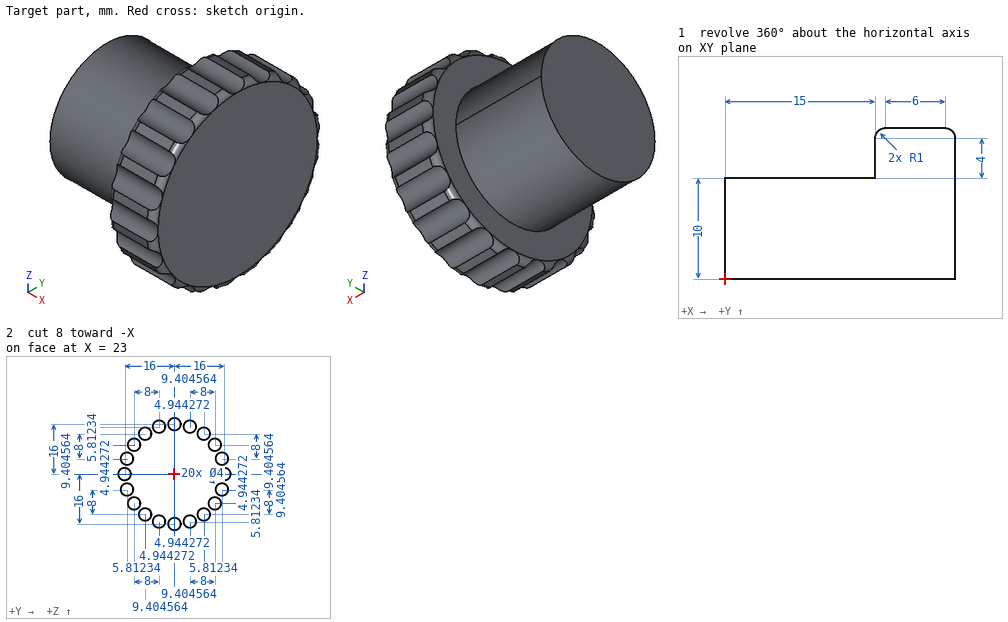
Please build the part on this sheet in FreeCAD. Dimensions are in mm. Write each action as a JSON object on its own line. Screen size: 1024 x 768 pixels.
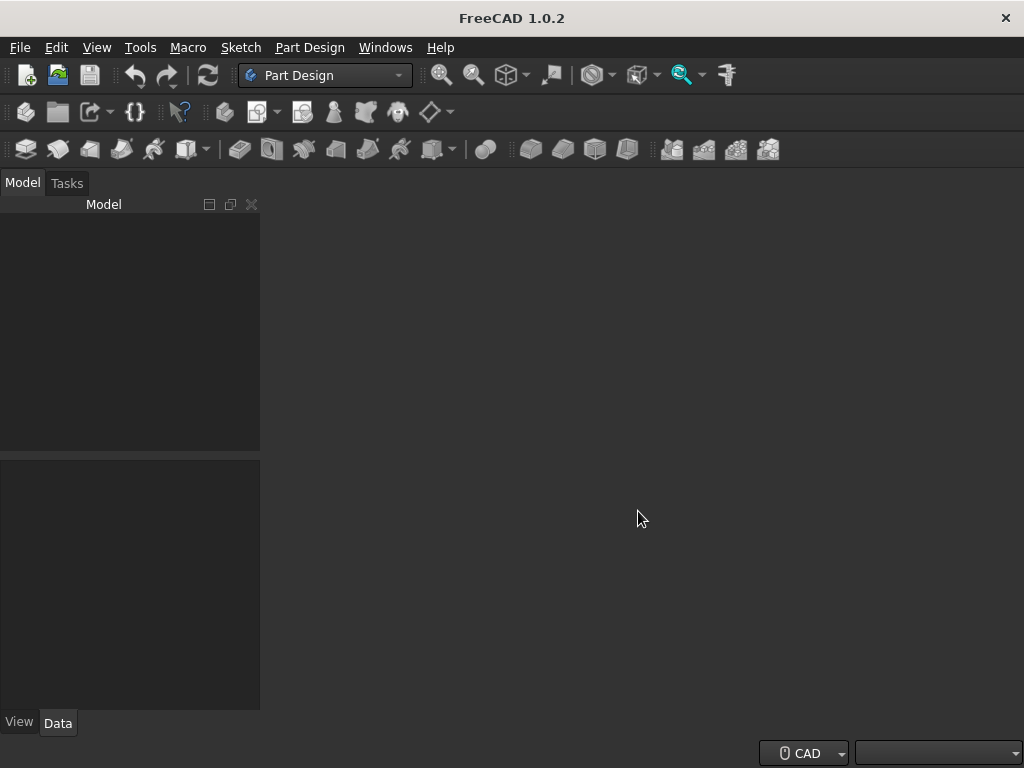
{"action": "left_click", "coordinate": [26, 76]}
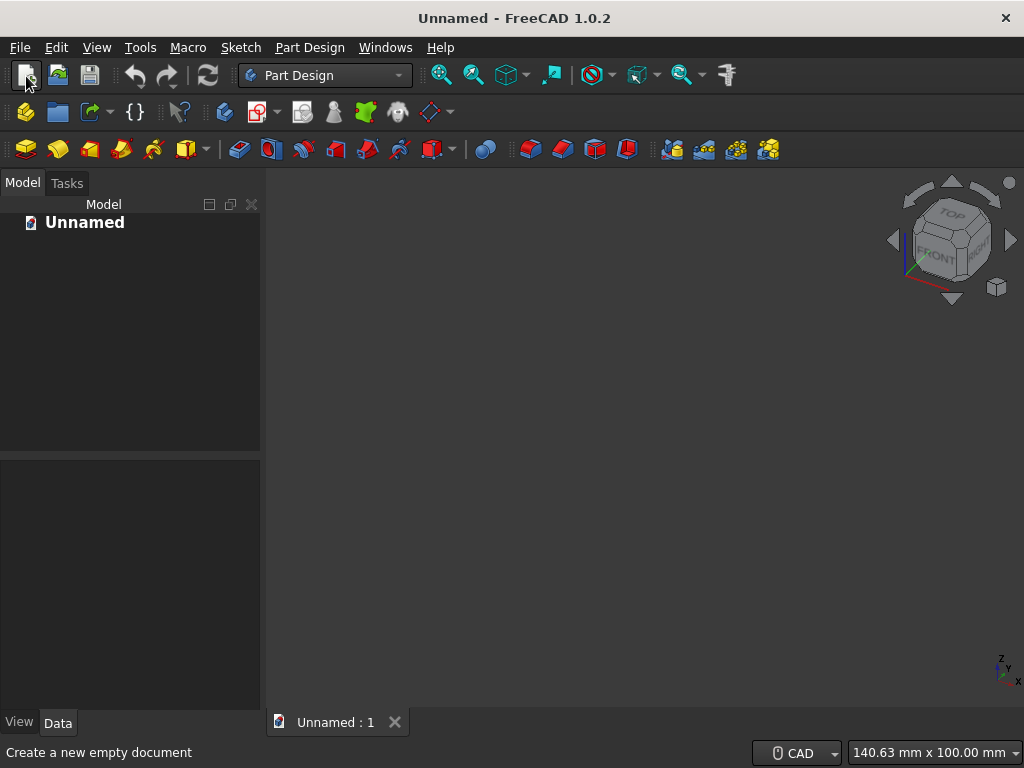
{"action": "left_click", "coordinate": [258, 112]}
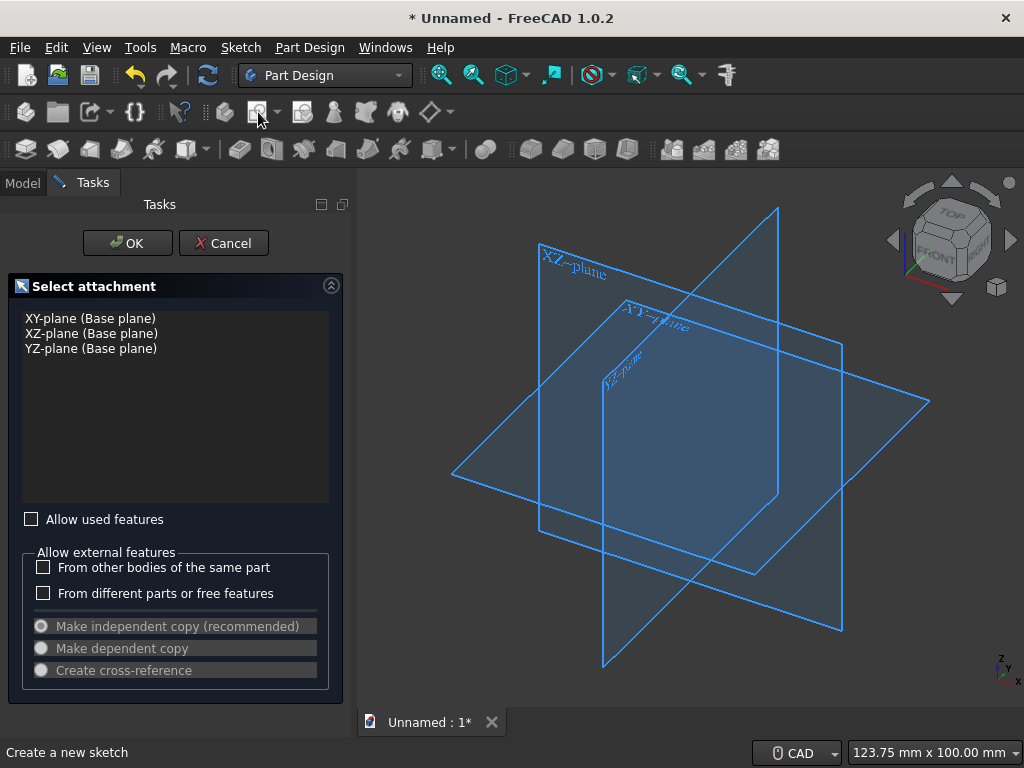
{"action": "left_click", "coordinate": [82, 318]}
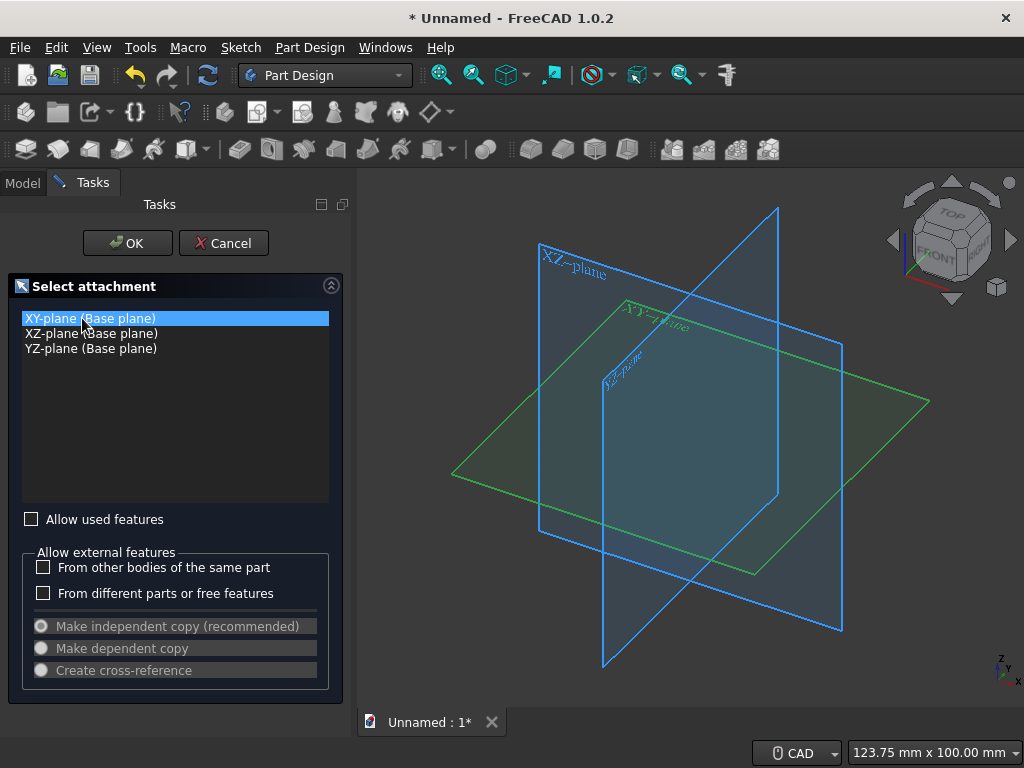
{"action": "left_click", "coordinate": [128, 243]}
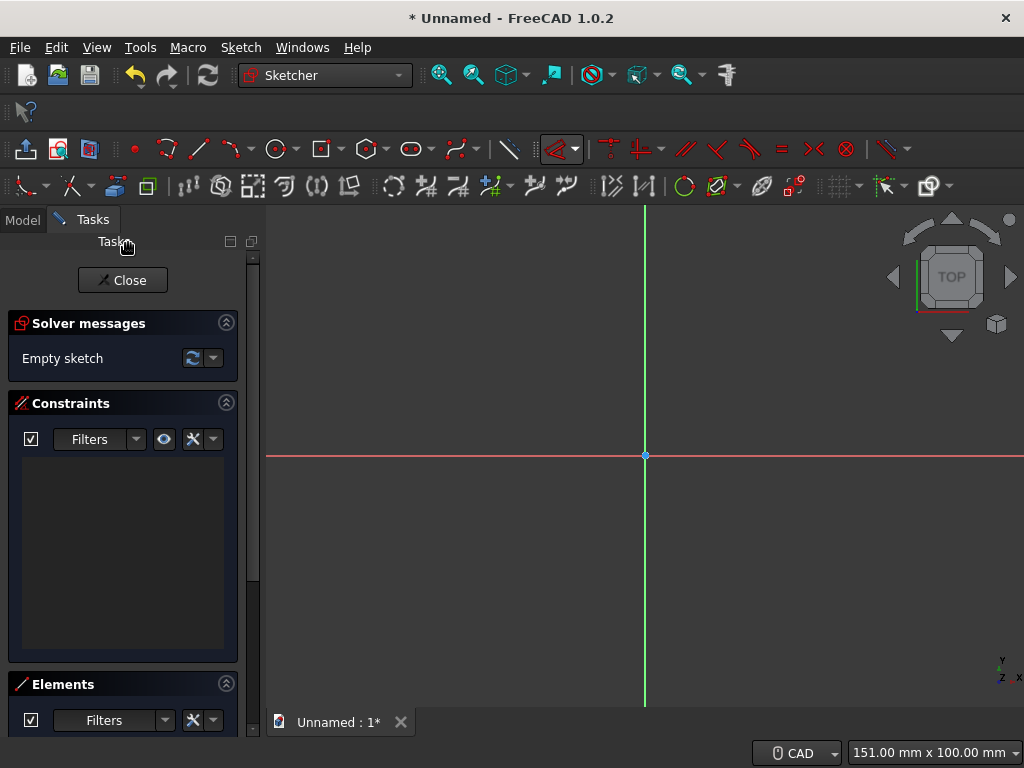
{"action": "scroll", "coordinate": [757, 402], "scroll_direction": "up", "scroll_amount": 6}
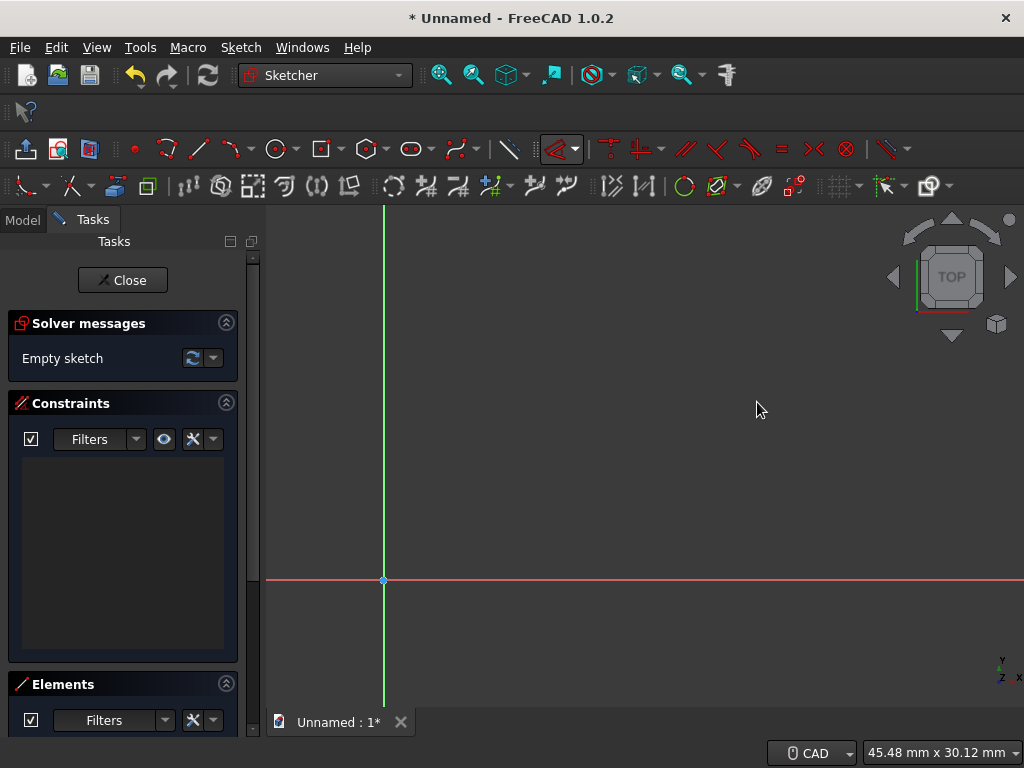
{"action": "left_click", "coordinate": [200, 150]}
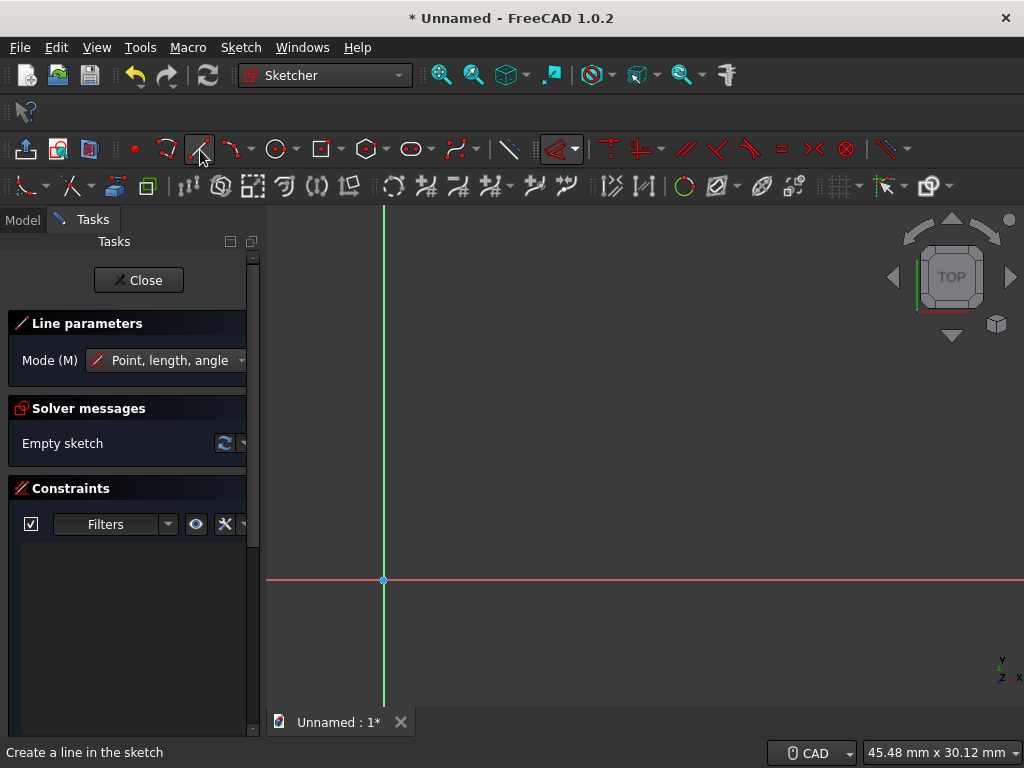
{"action": "left_click", "coordinate": [750, 330]}
{"action": "left_click", "coordinate": [650, 330]}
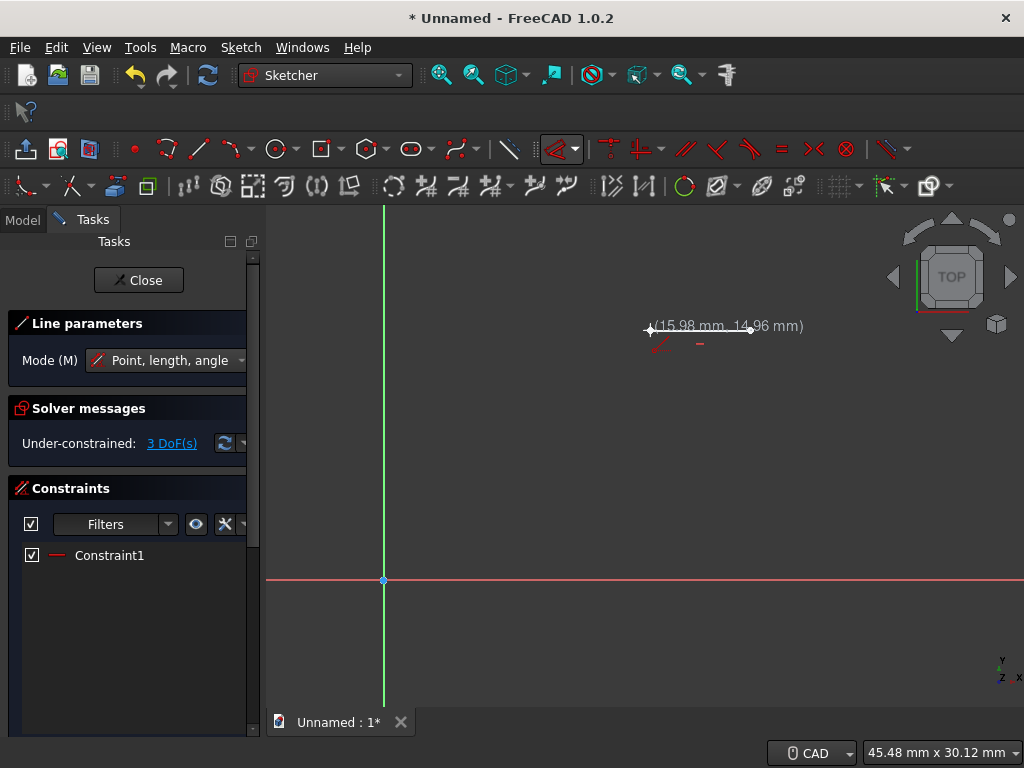
{"action": "left_click", "coordinate": [168, 150]}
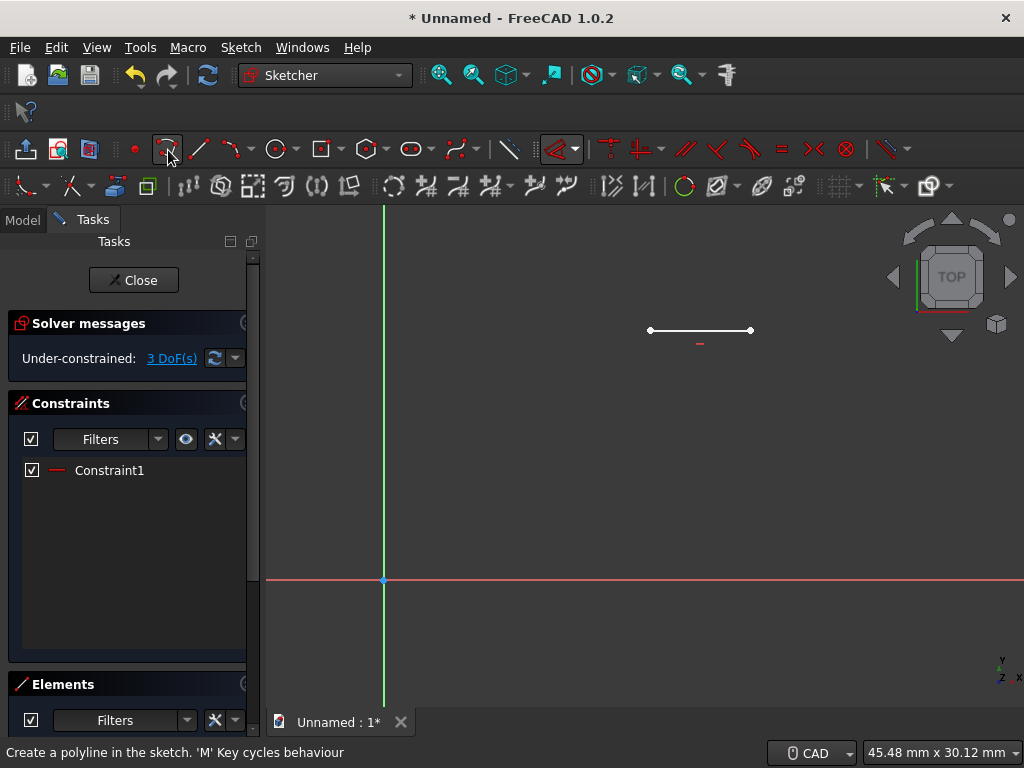
{"action": "left_click", "coordinate": [634, 347]}
{"action": "left_click", "coordinate": [634, 414]}
{"action": "left_click", "coordinate": [384, 414]}
{"action": "left_click", "coordinate": [384, 580]}
{"action": "left_click", "coordinate": [767, 571]}
{"action": "left_click", "coordinate": [767, 347]}
{"action": "right_click", "coordinate": [767, 347]}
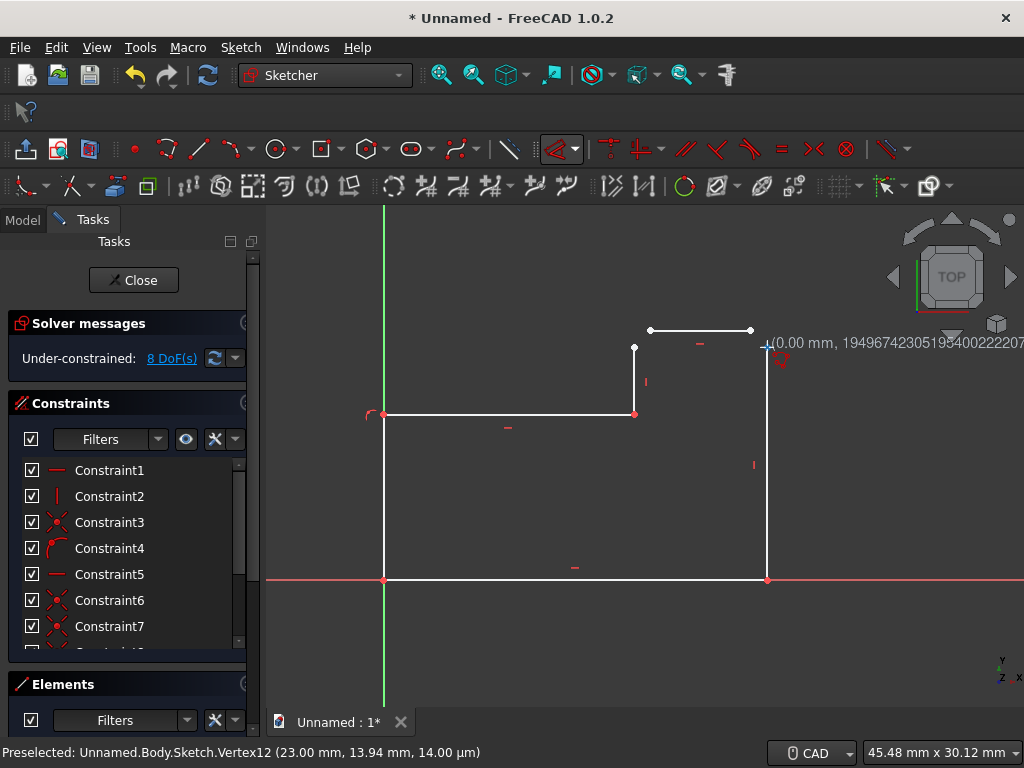
{"action": "left_click", "coordinate": [232, 150]}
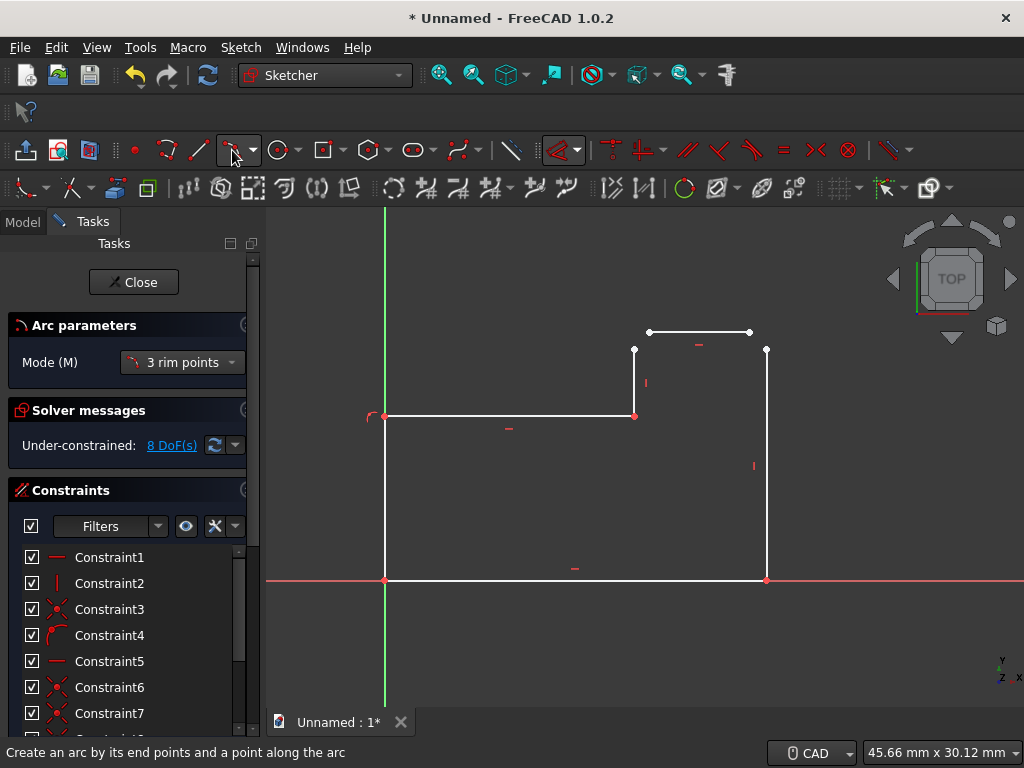
{"action": "left_click", "coordinate": [650, 332]}
{"action": "left_click", "coordinate": [634, 349]}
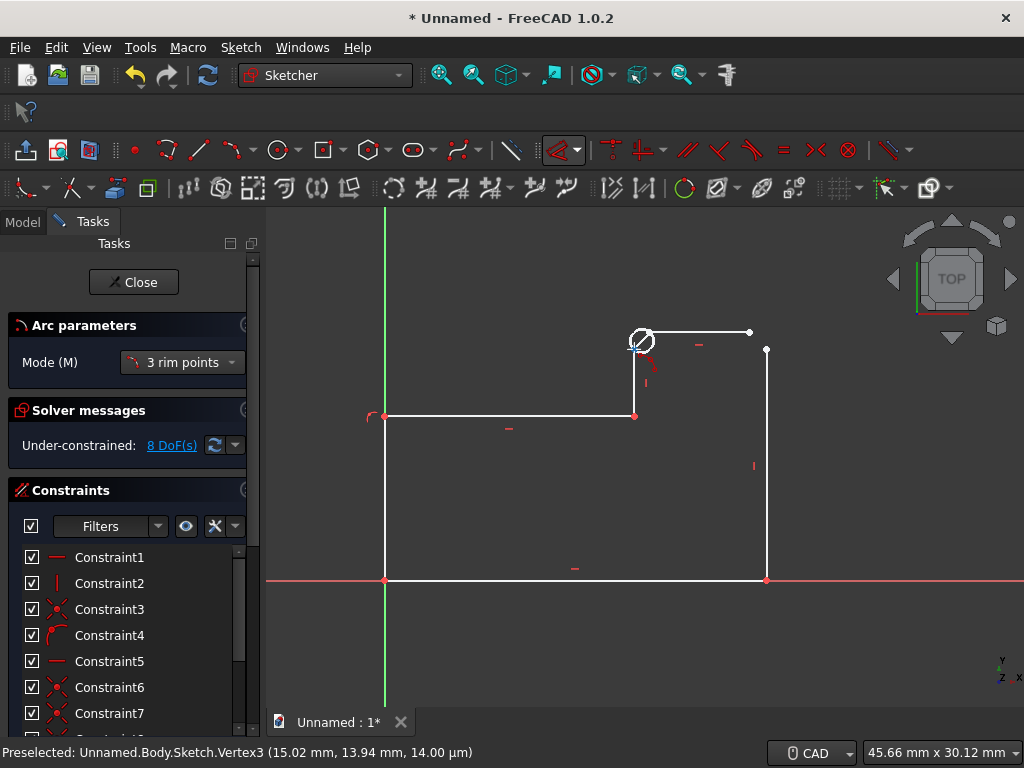
{"action": "scroll", "coordinate": [639, 337], "scroll_direction": "up", "scroll_amount": 6}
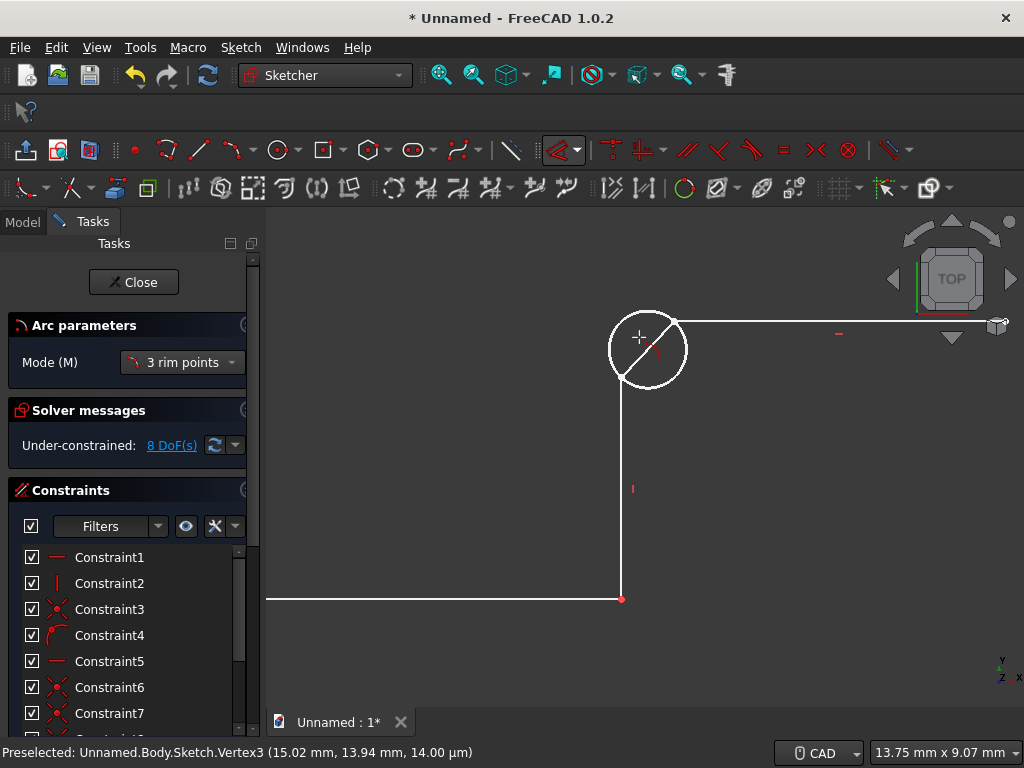
{"action": "left_click", "coordinate": [636, 336]}